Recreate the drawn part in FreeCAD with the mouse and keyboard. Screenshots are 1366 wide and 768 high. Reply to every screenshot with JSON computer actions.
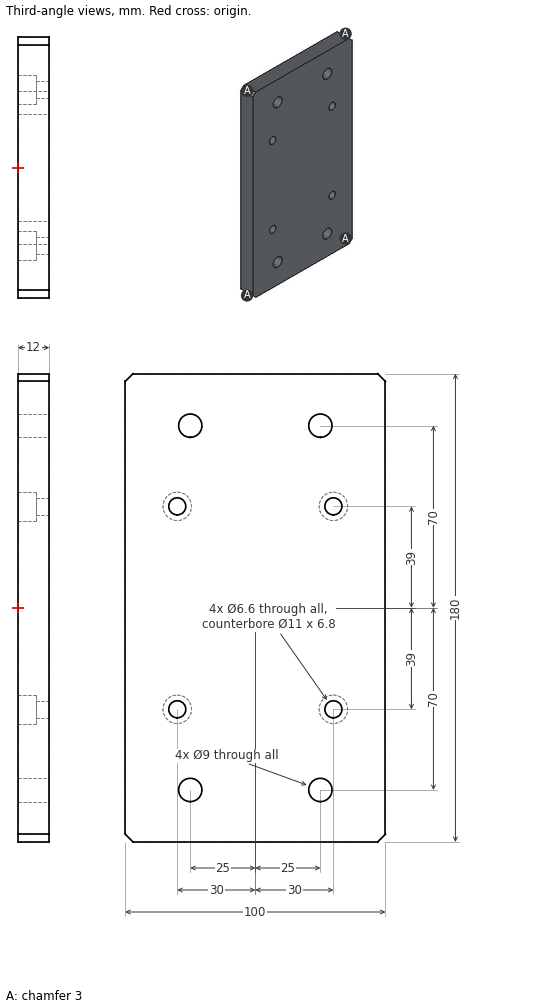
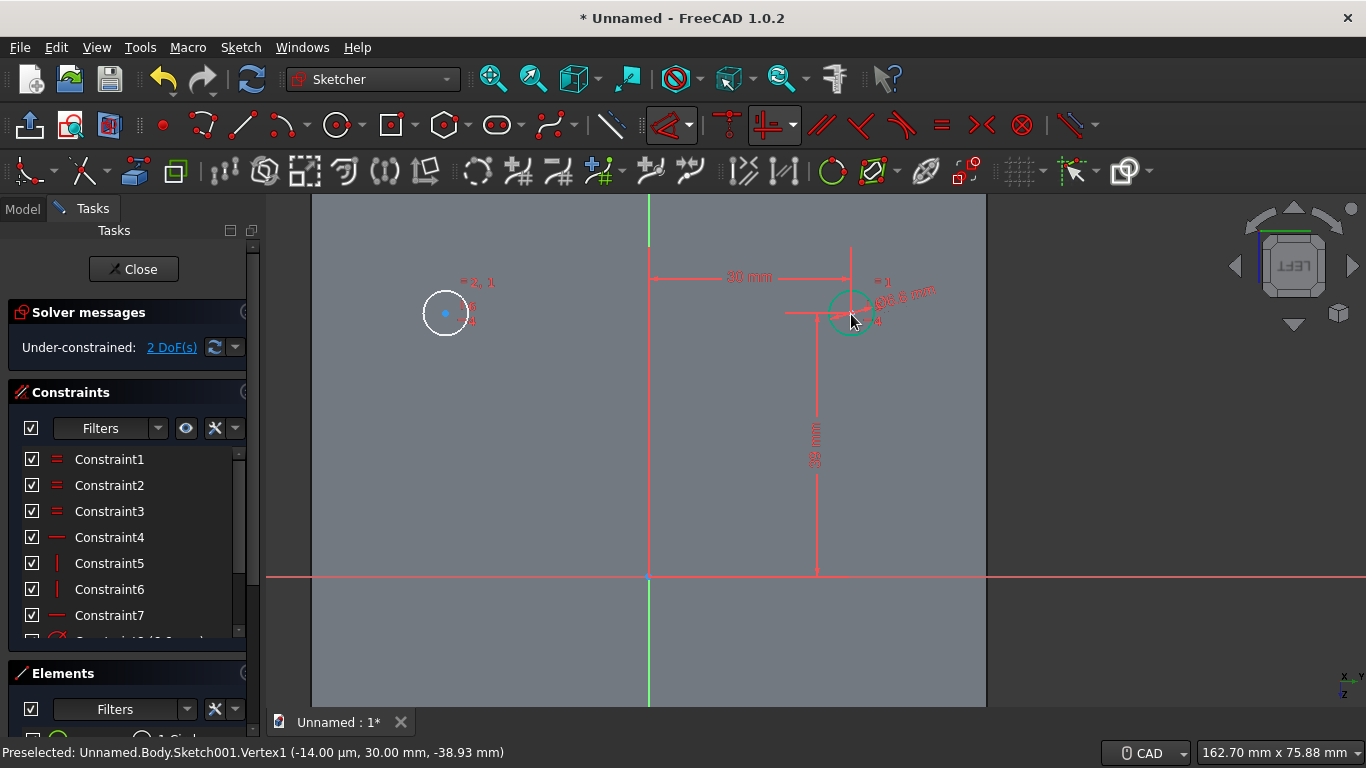
{"action": "left_click", "coordinate": [446, 313]}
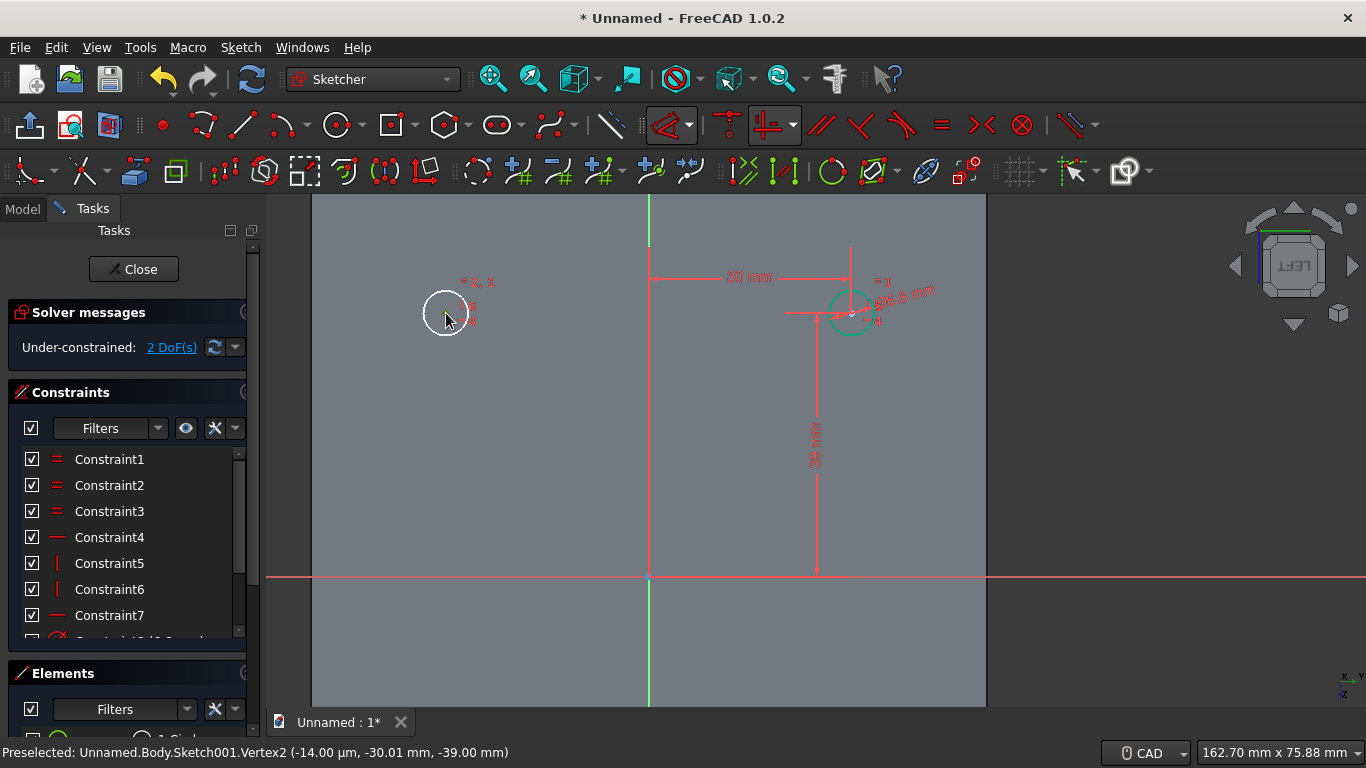
{"action": "left_click", "coordinate": [692, 126]}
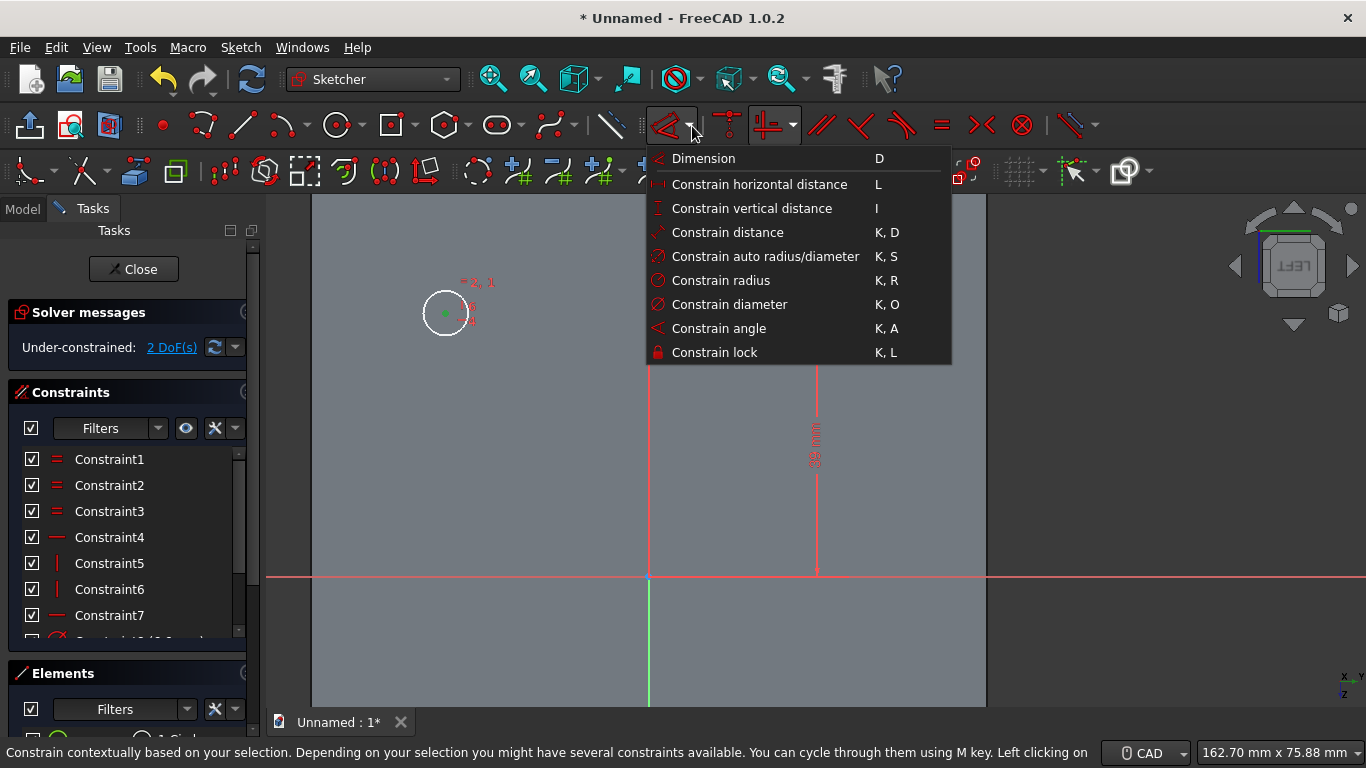
{"action": "left_click", "coordinate": [799, 184]}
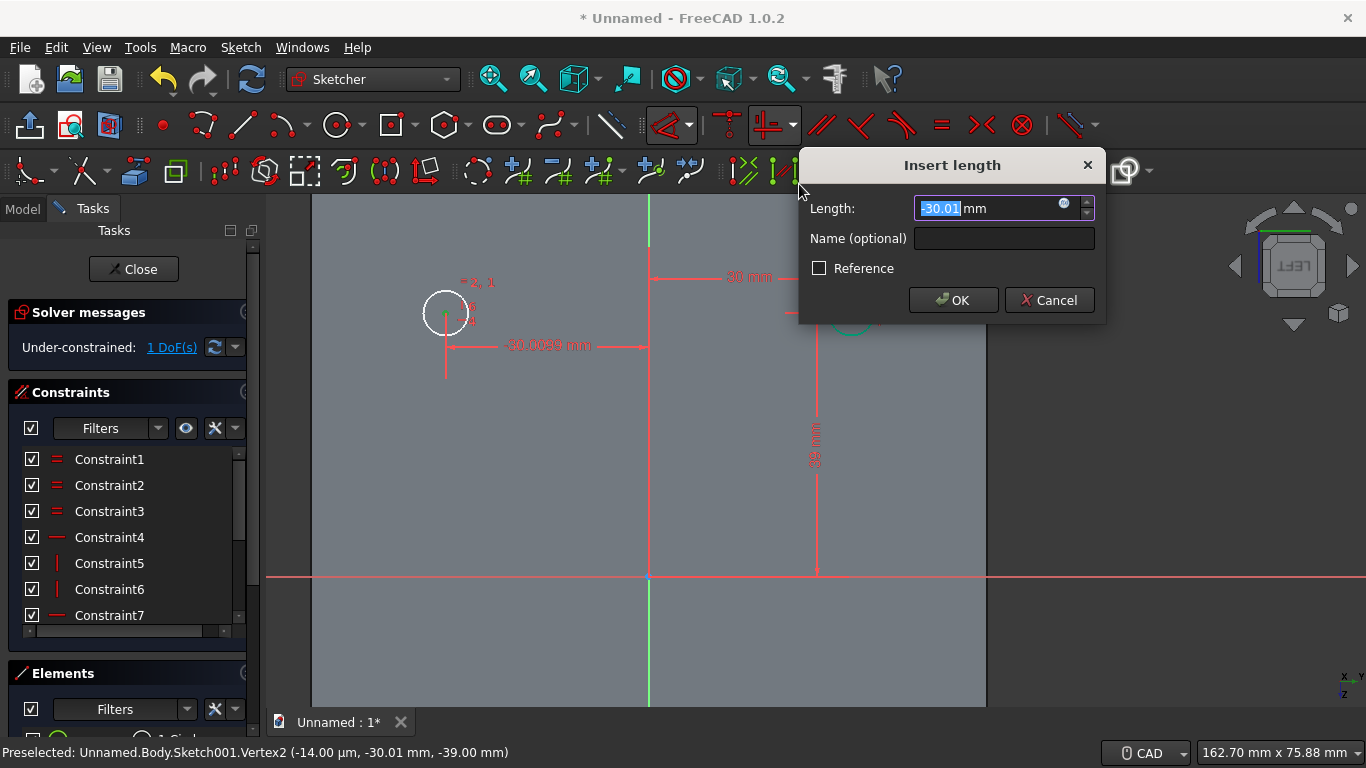
{"action": "type", "text": "-30"}
{"action": "key", "text": "Return"}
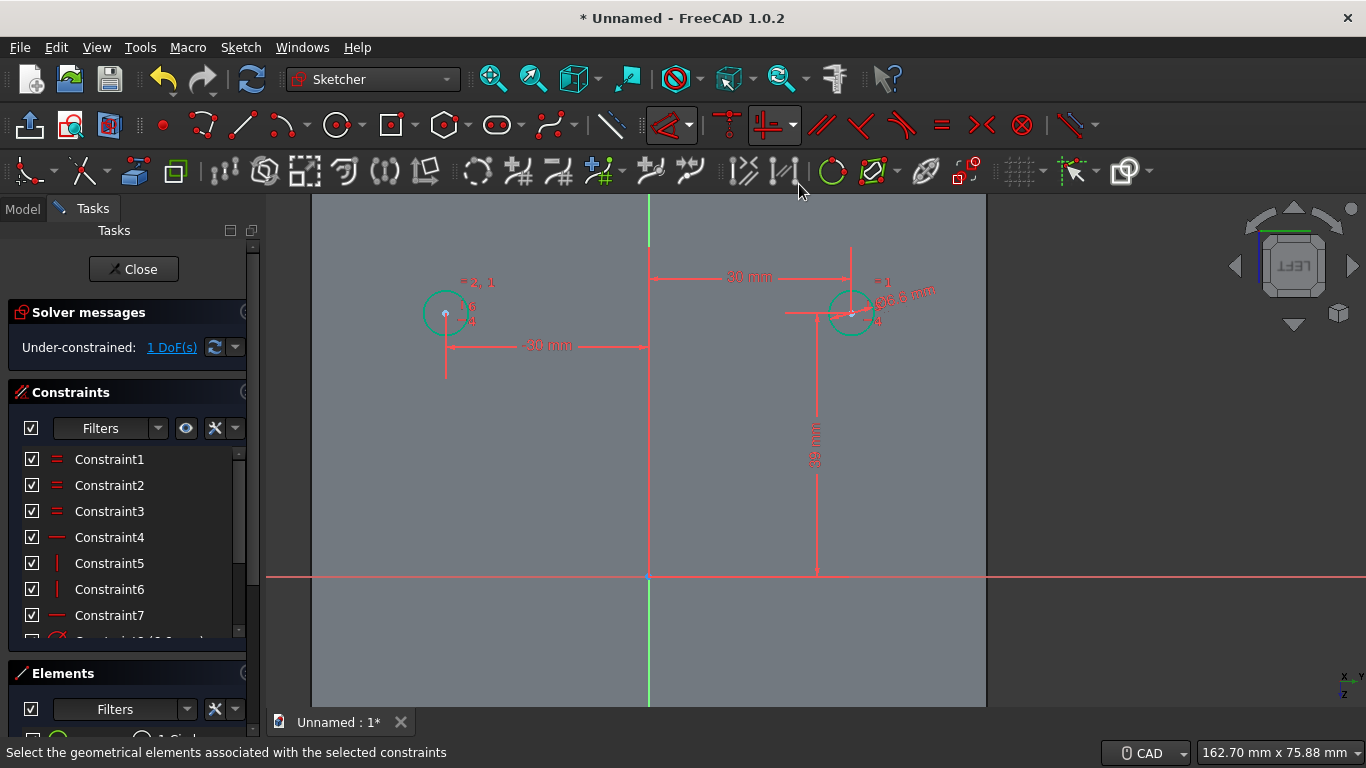
{"action": "scroll", "coordinate": [868, 297], "scroll_direction": "down", "scroll_amount": 3}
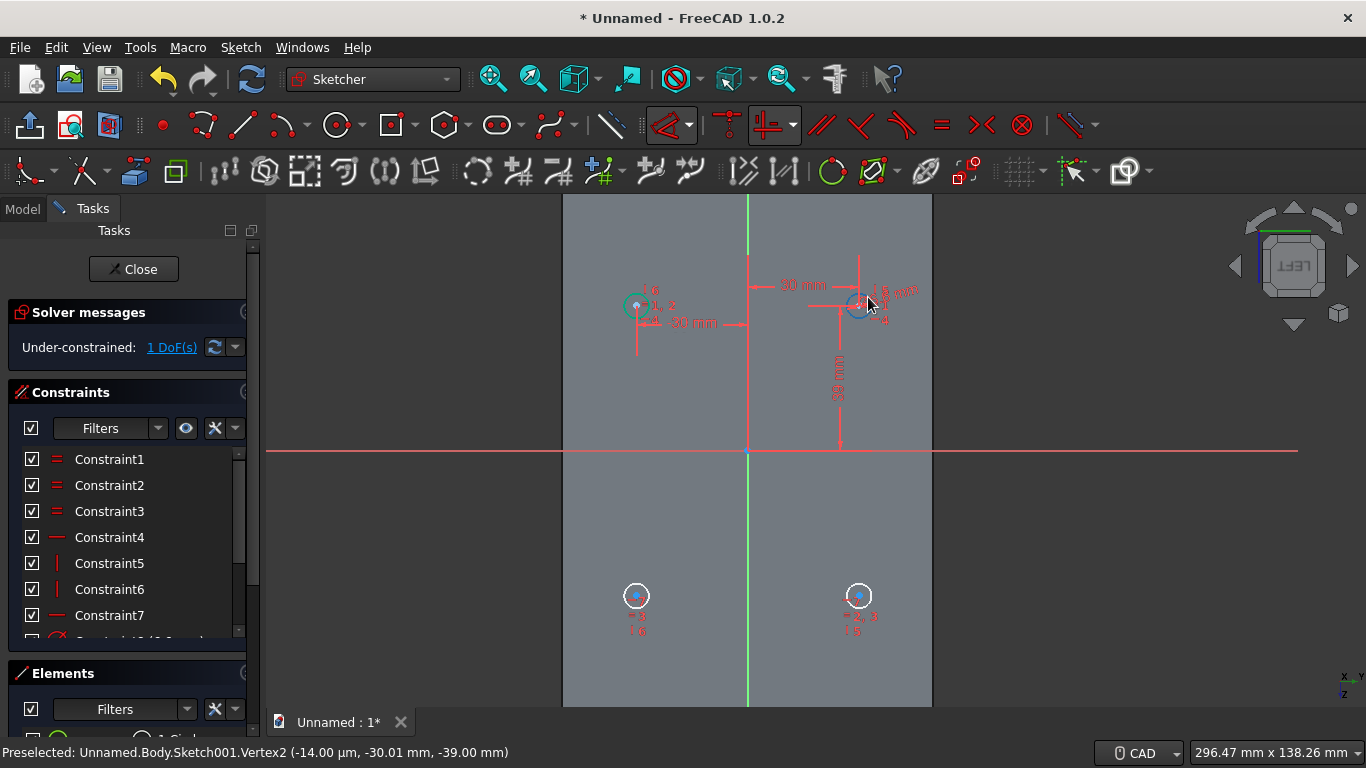
{"action": "left_click", "coordinate": [859, 596]}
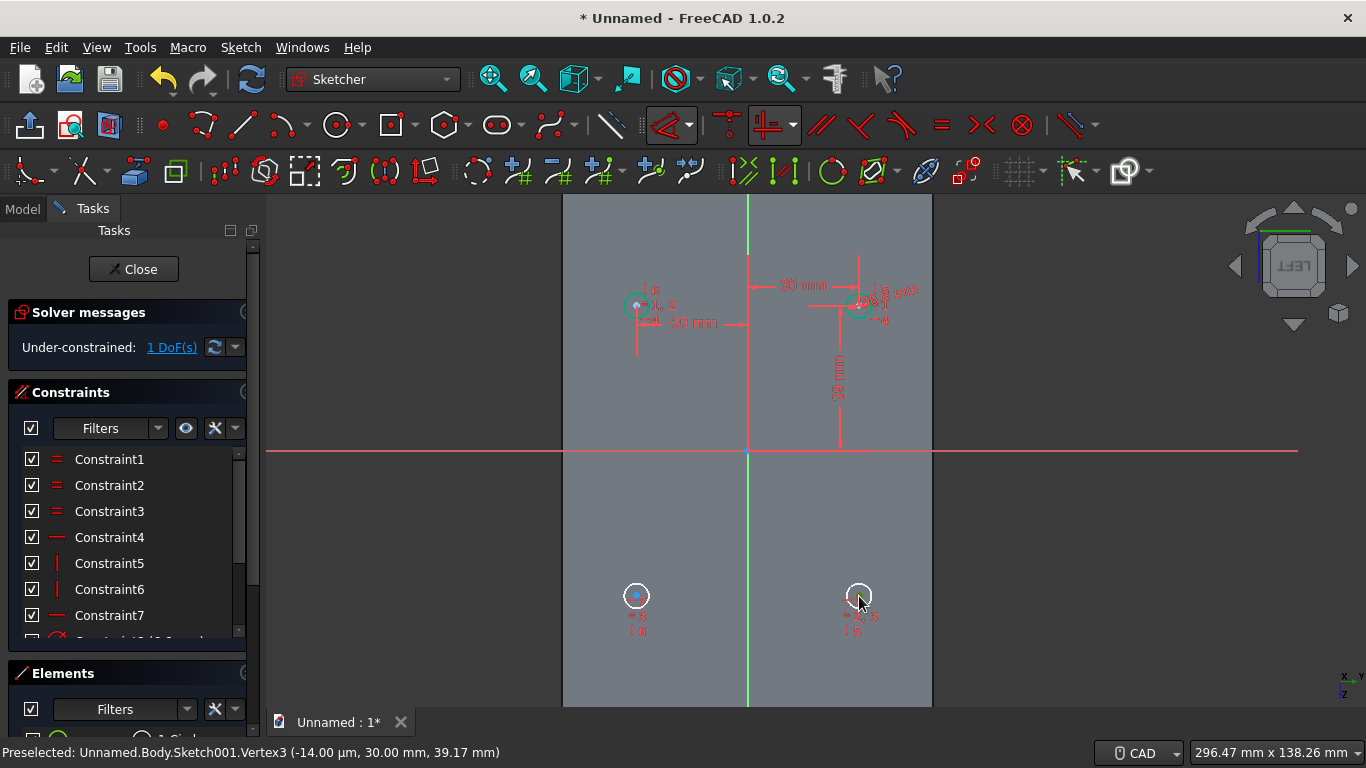
{"action": "left_click", "coordinate": [692, 126]}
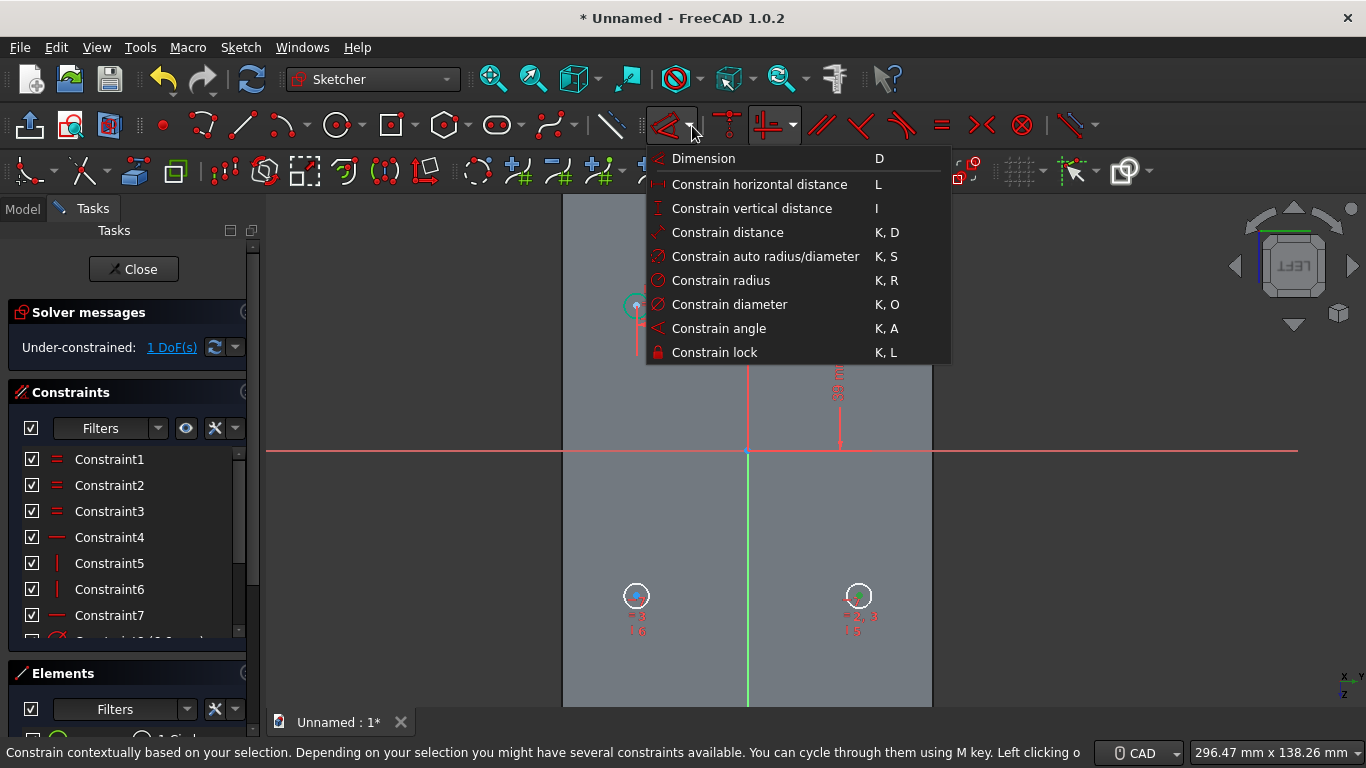
{"action": "left_click", "coordinate": [799, 208]}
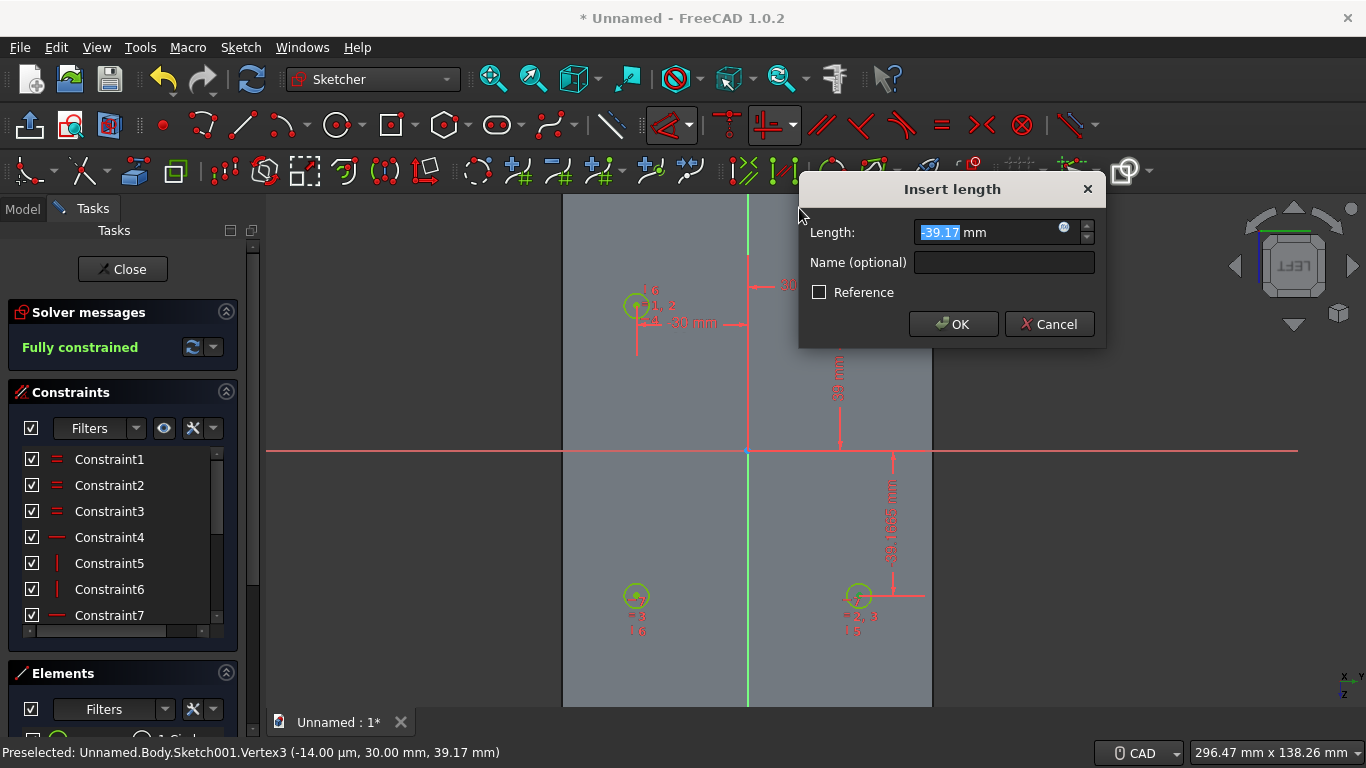
{"action": "type", "text": "-39"}
{"action": "key", "text": "Return"}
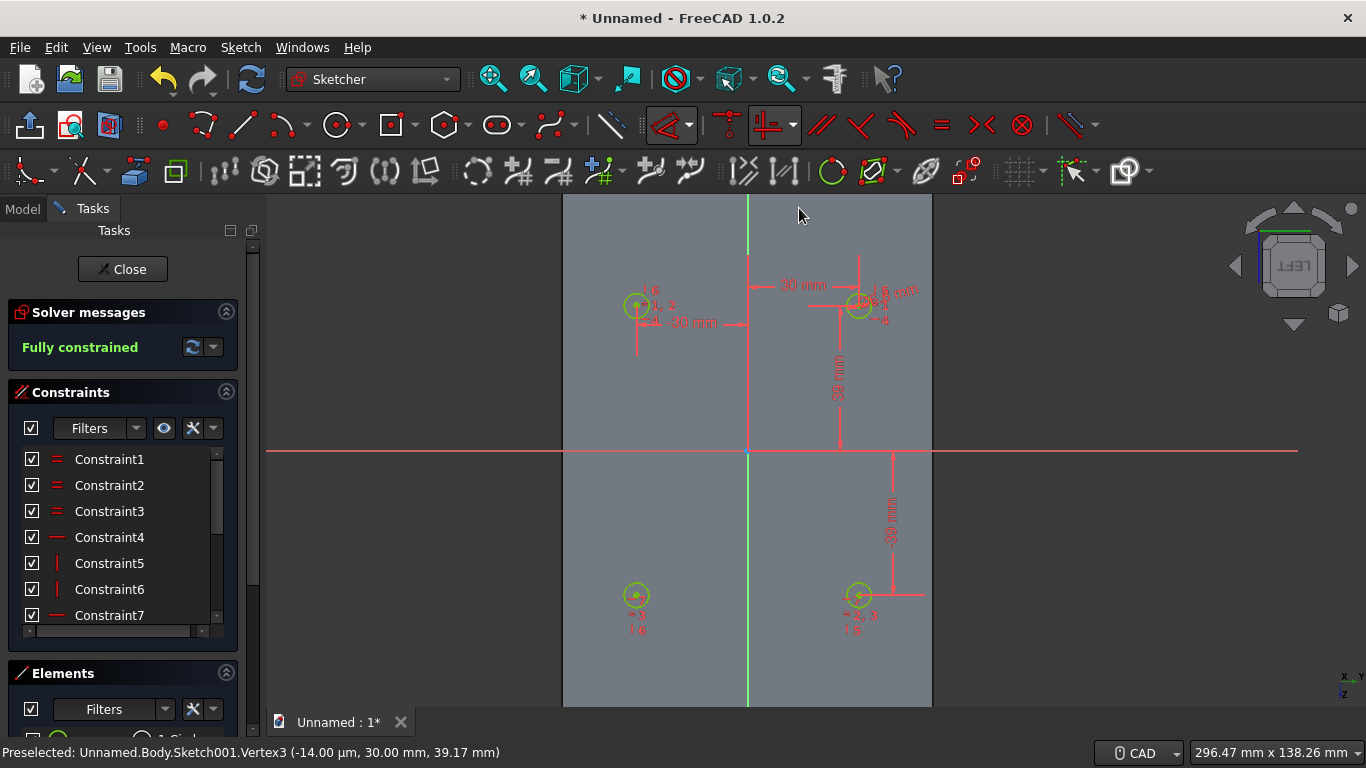
{"action": "left_click", "coordinate": [123, 269]}